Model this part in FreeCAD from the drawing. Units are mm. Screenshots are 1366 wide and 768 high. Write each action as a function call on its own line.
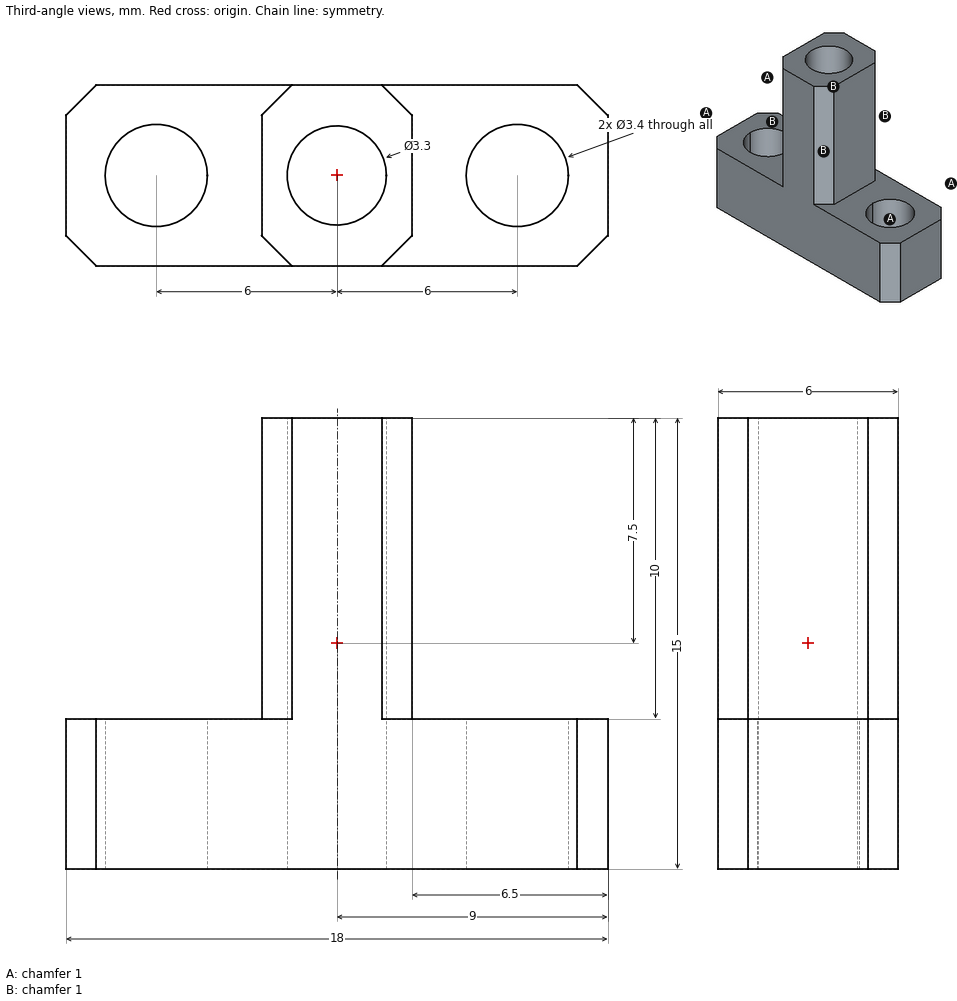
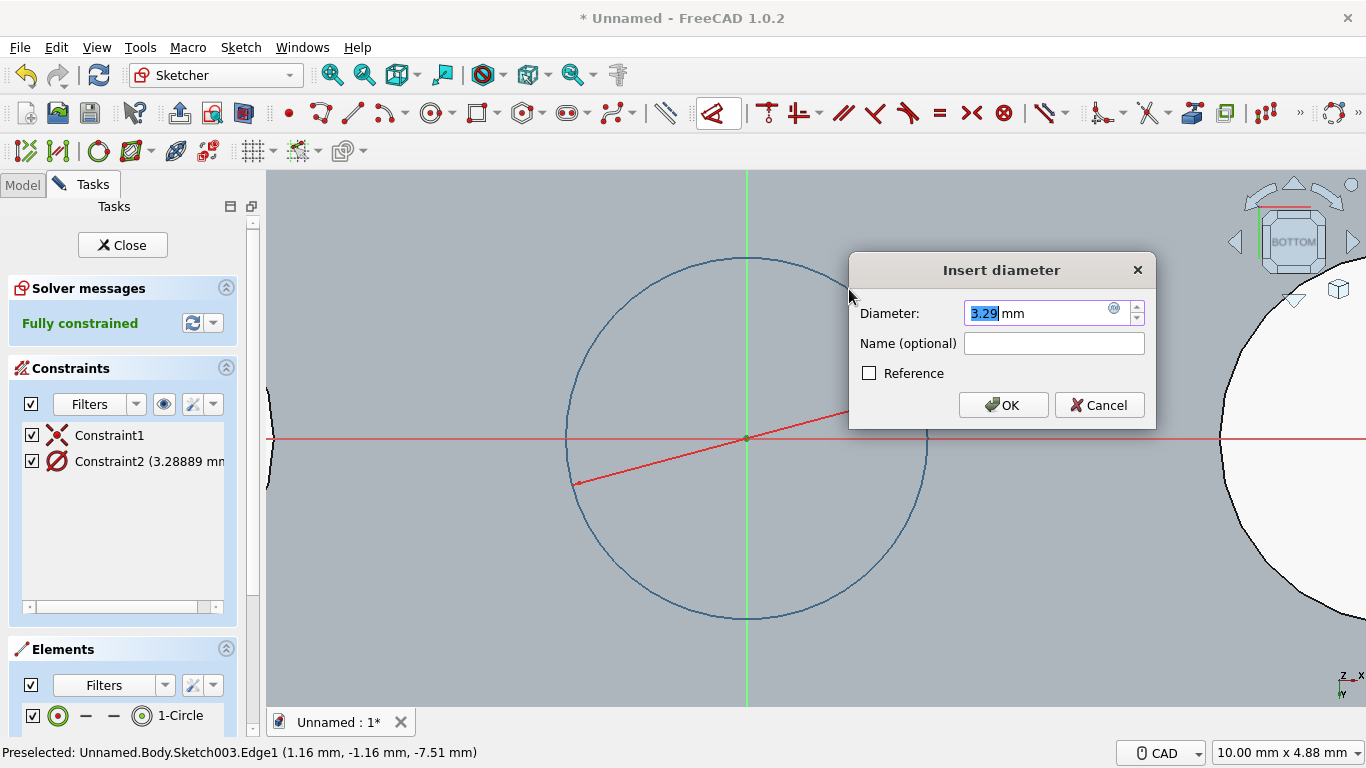
text(3.3)
key(Return)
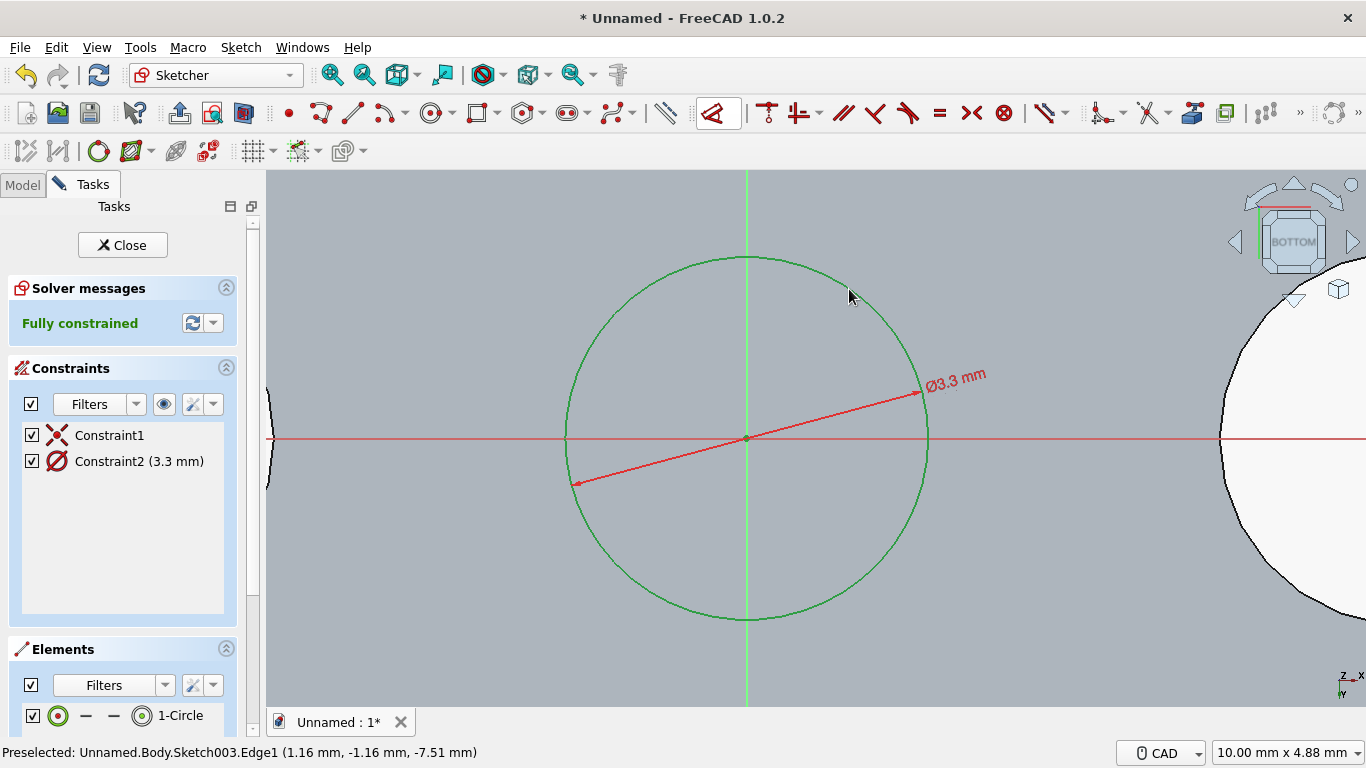
click(123, 245)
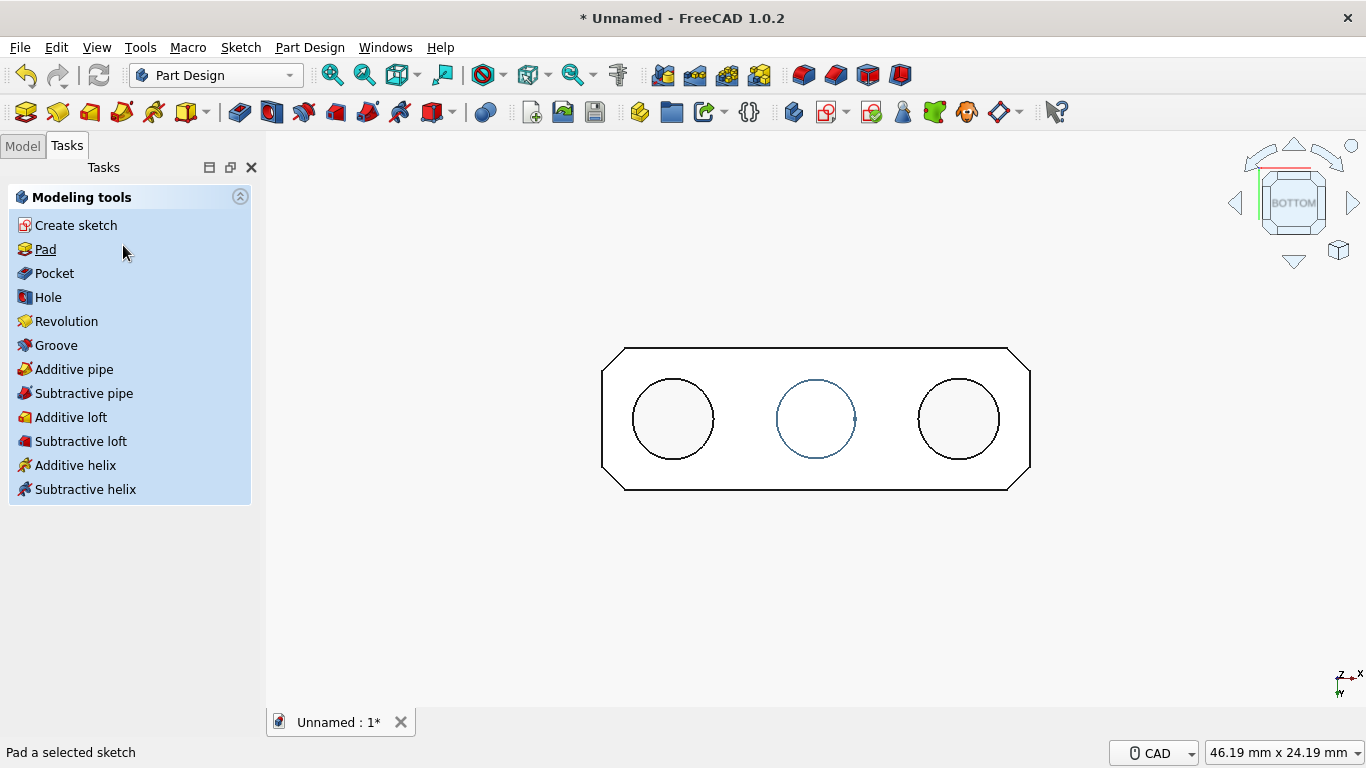
click(240, 112)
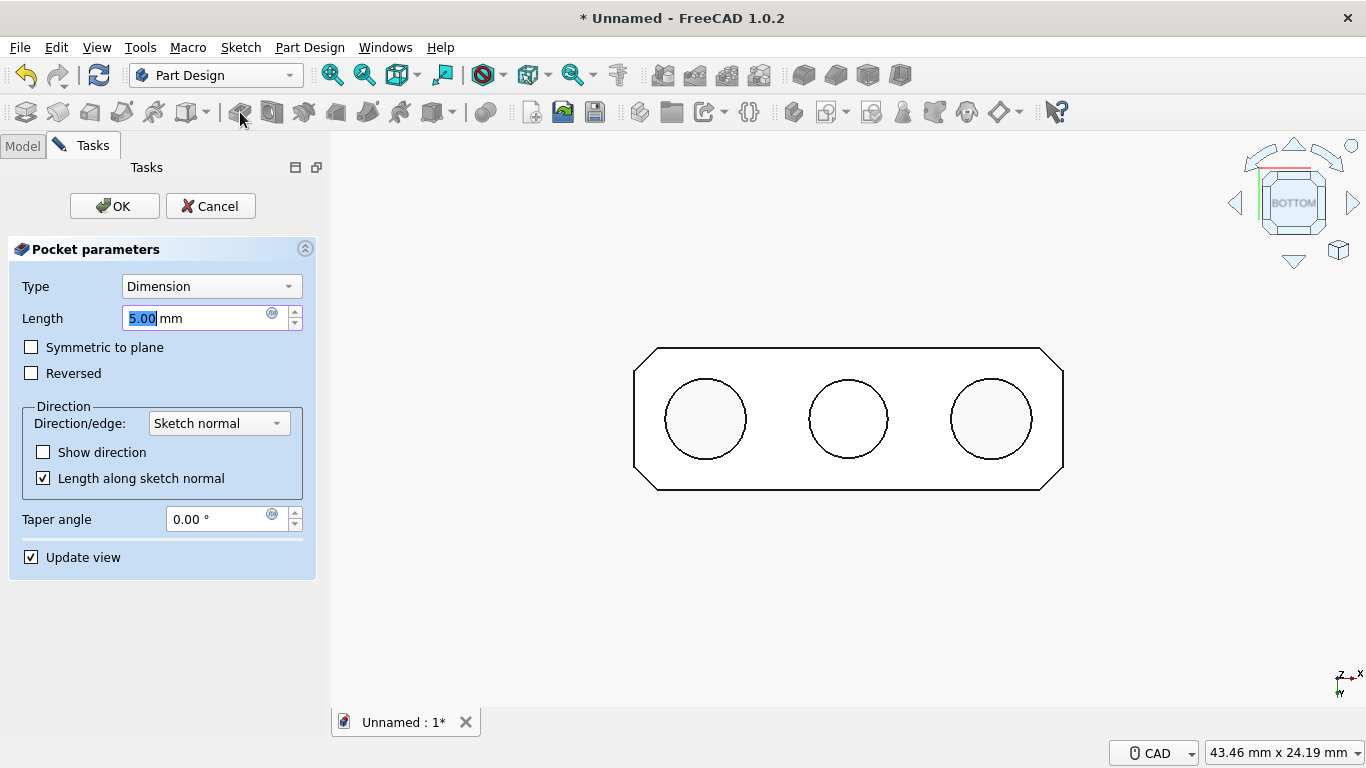
click(212, 286)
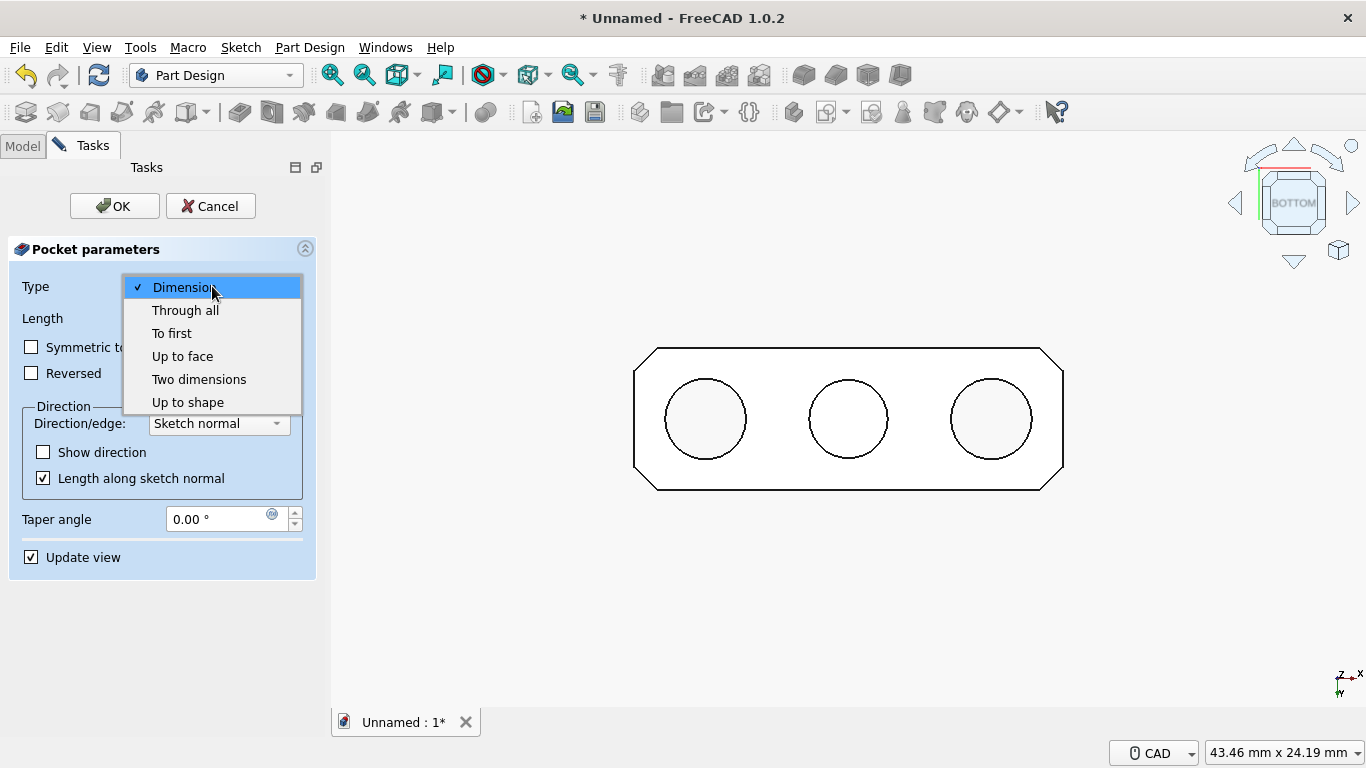
click(212, 310)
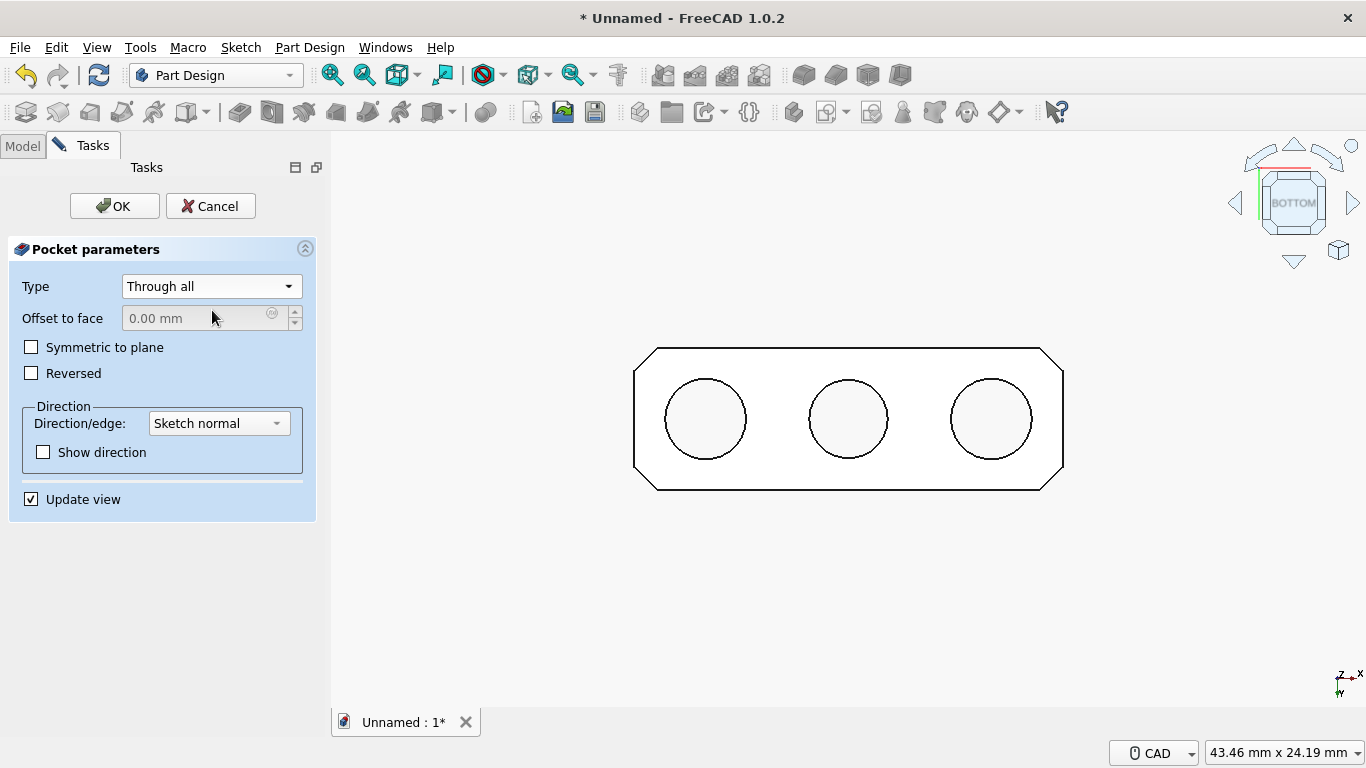
click(115, 206)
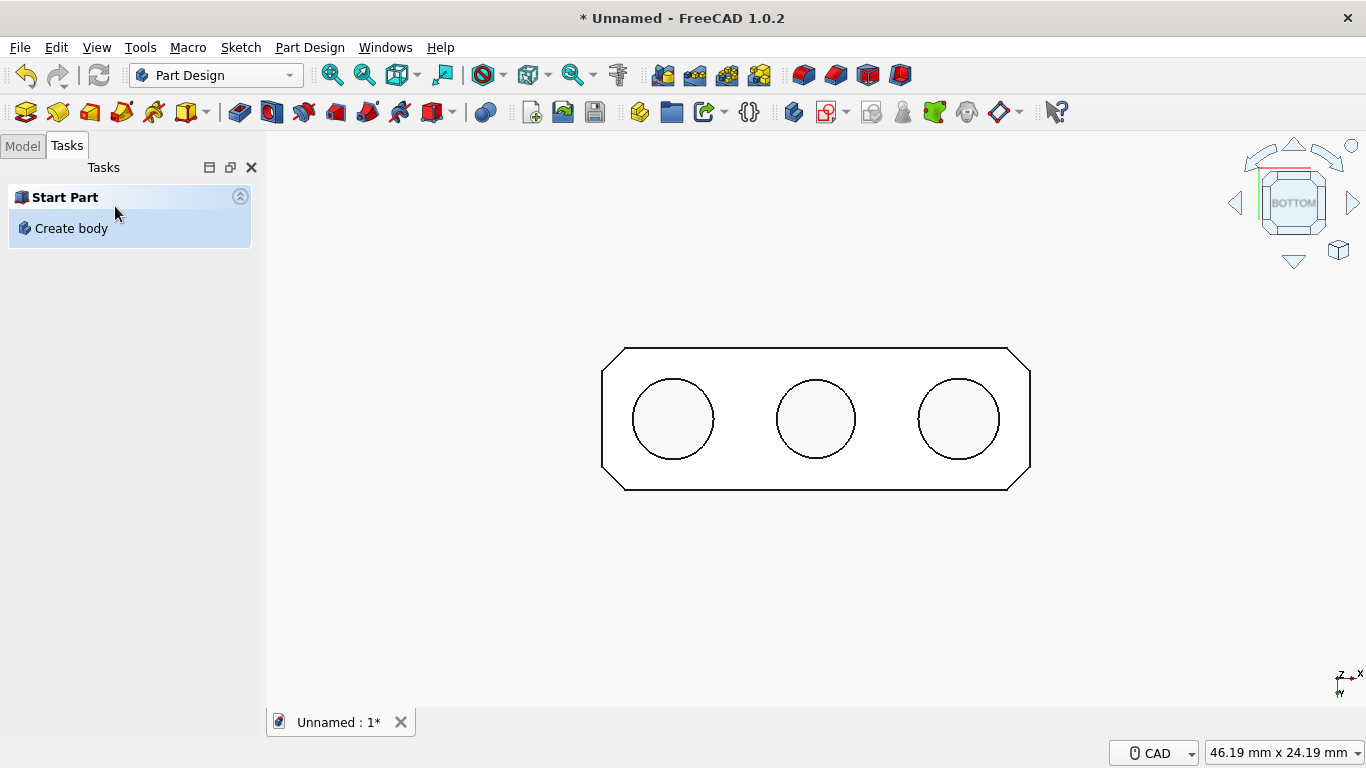
click(334, 76)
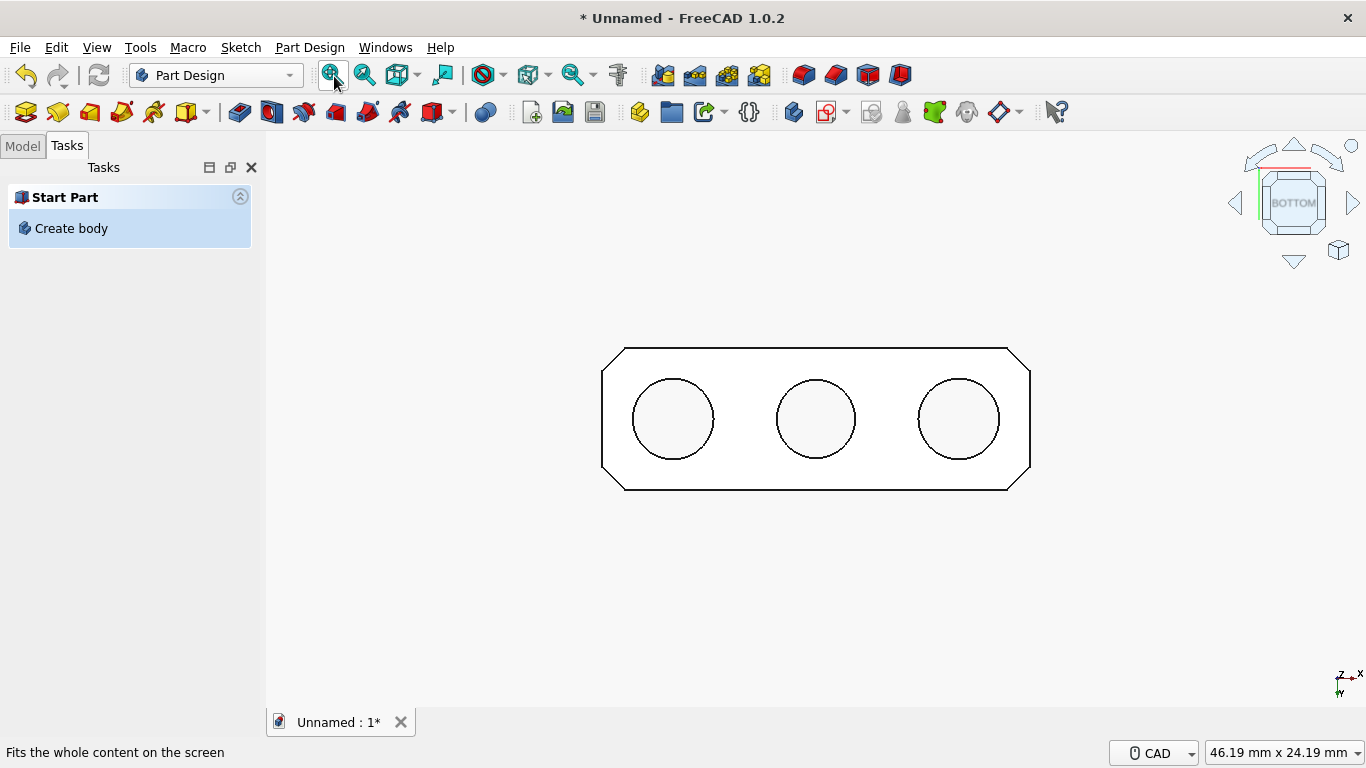
key(0)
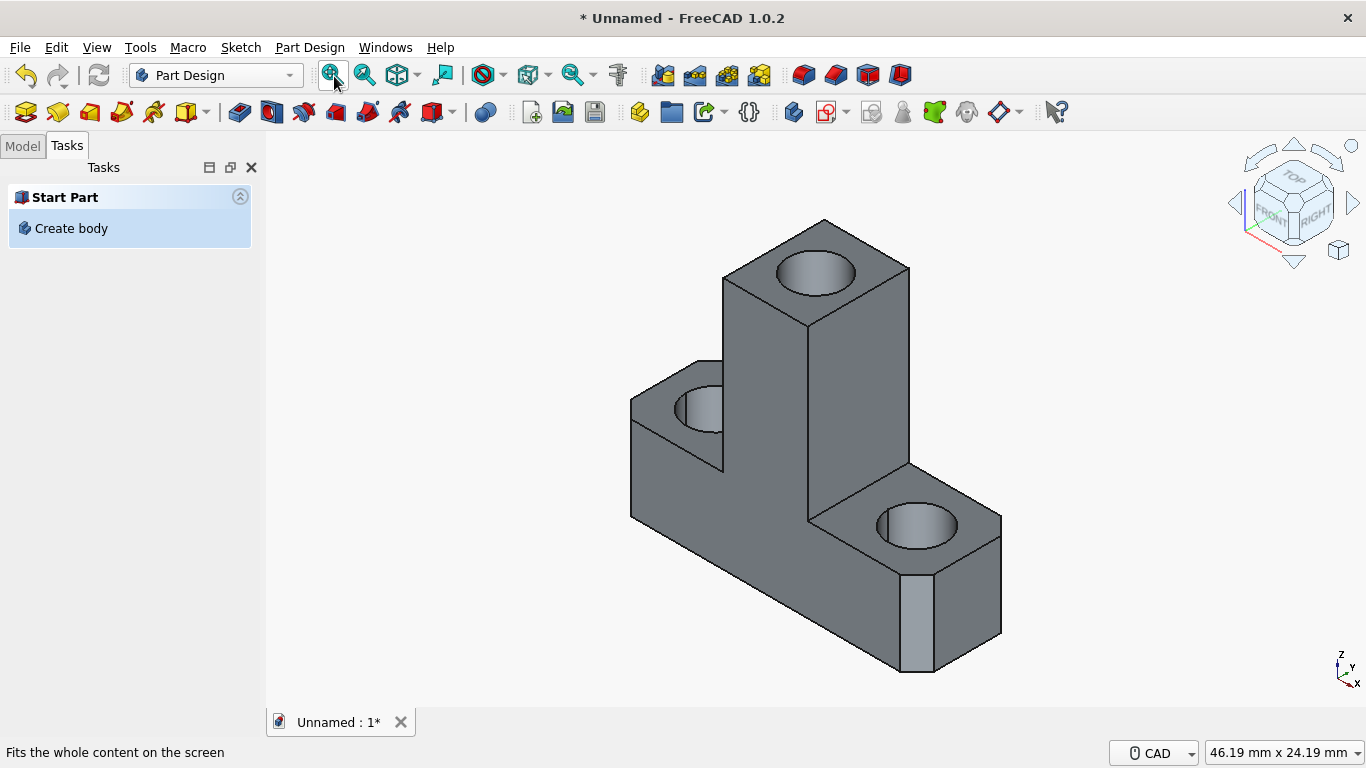
click(808, 423)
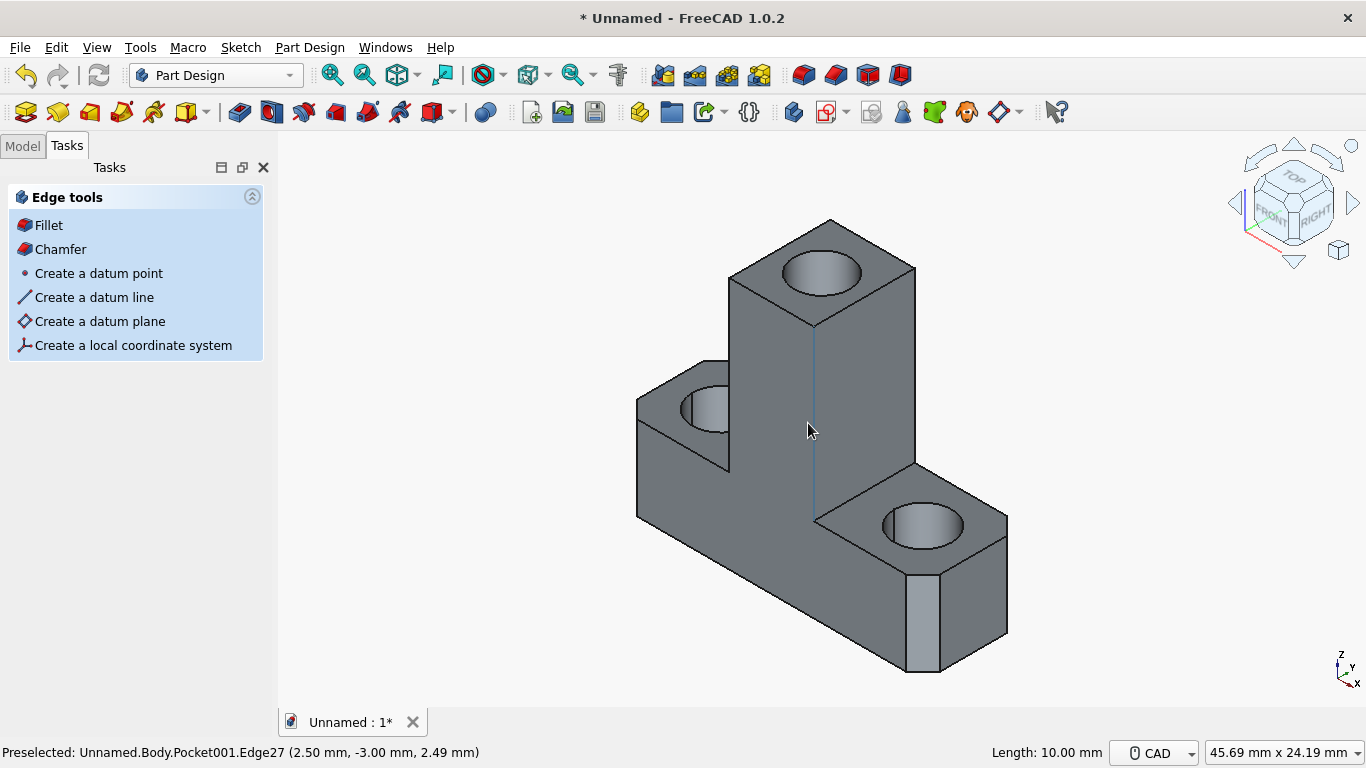
key(2)